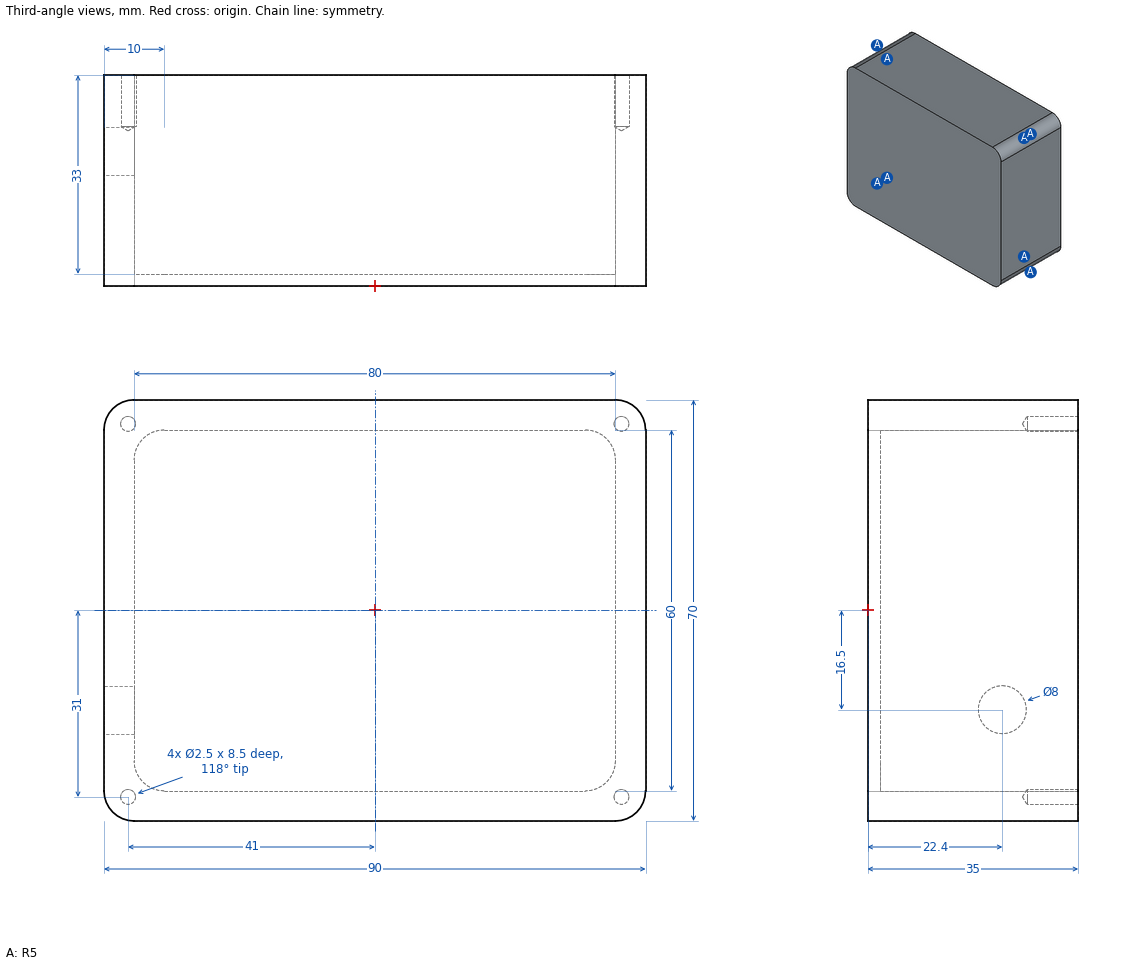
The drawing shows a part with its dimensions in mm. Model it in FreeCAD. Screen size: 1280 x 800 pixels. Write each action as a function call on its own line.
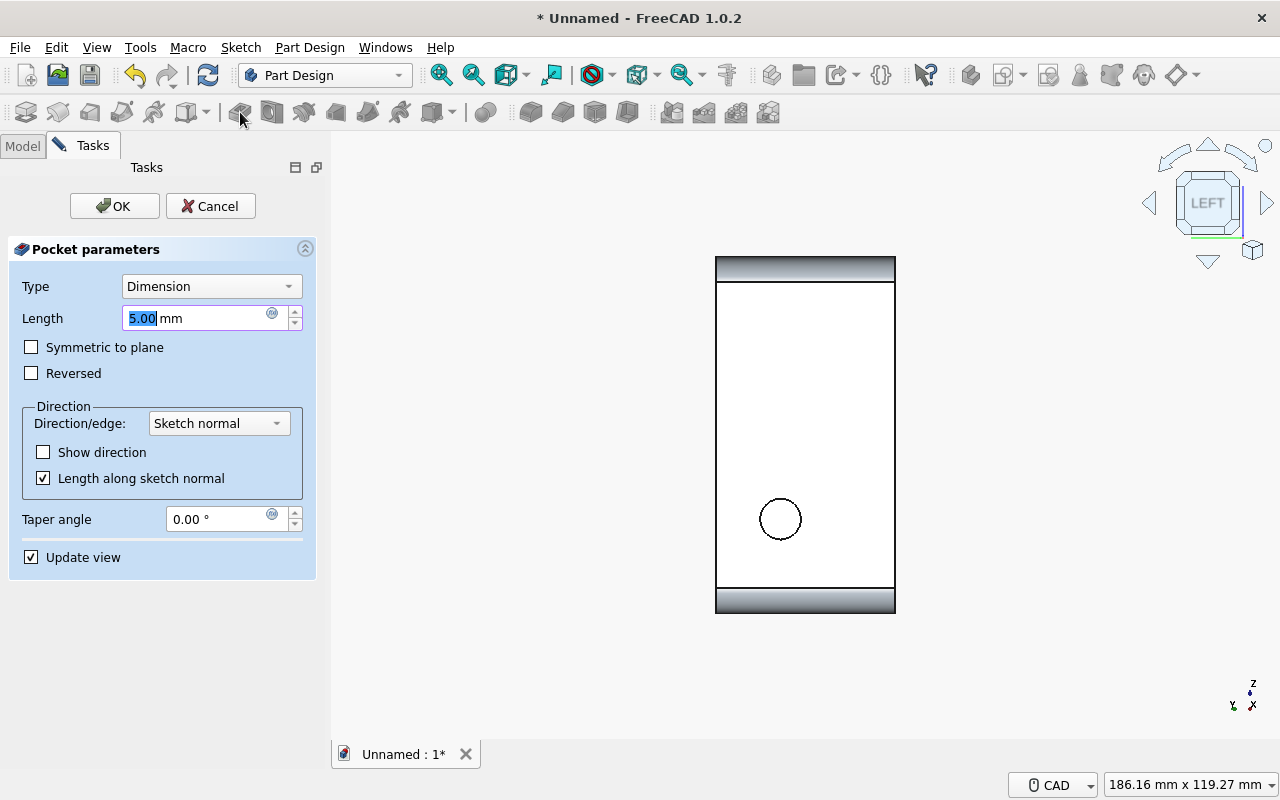
text(10)
key(Tab)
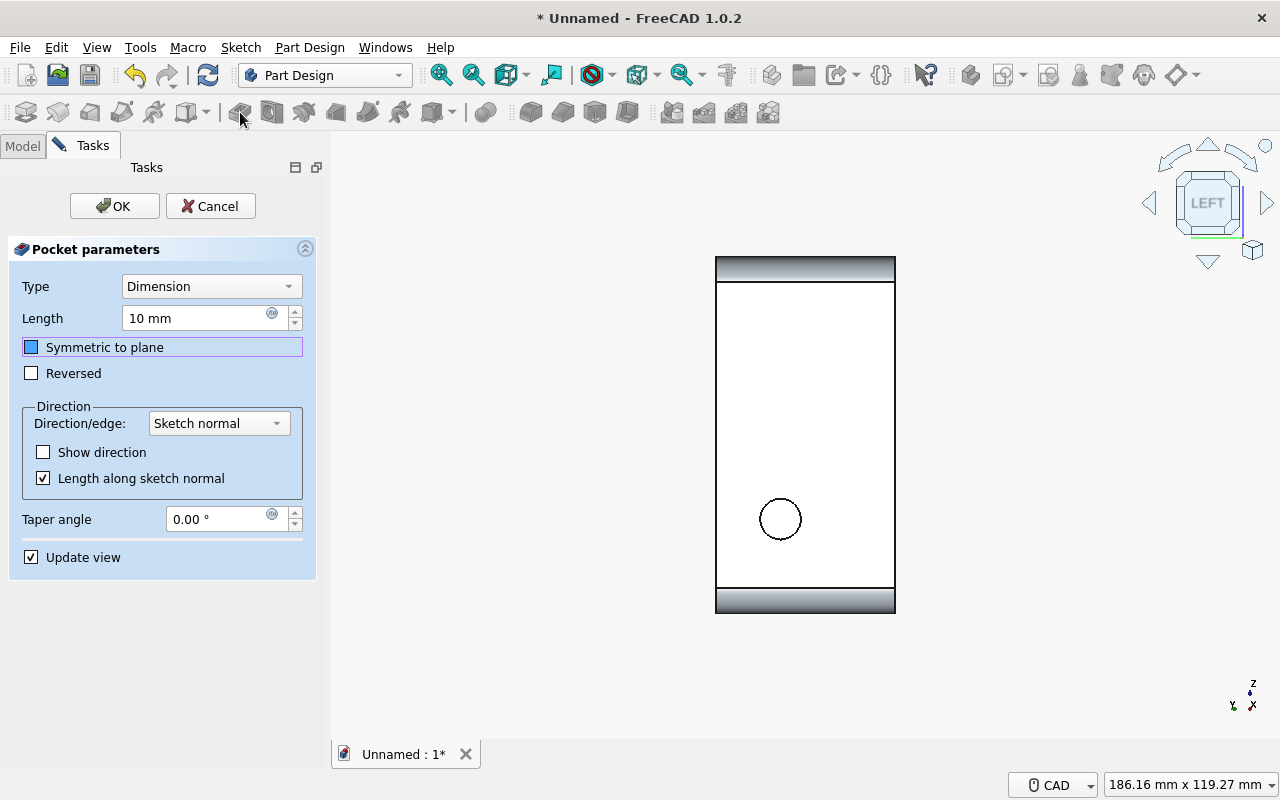
click(115, 206)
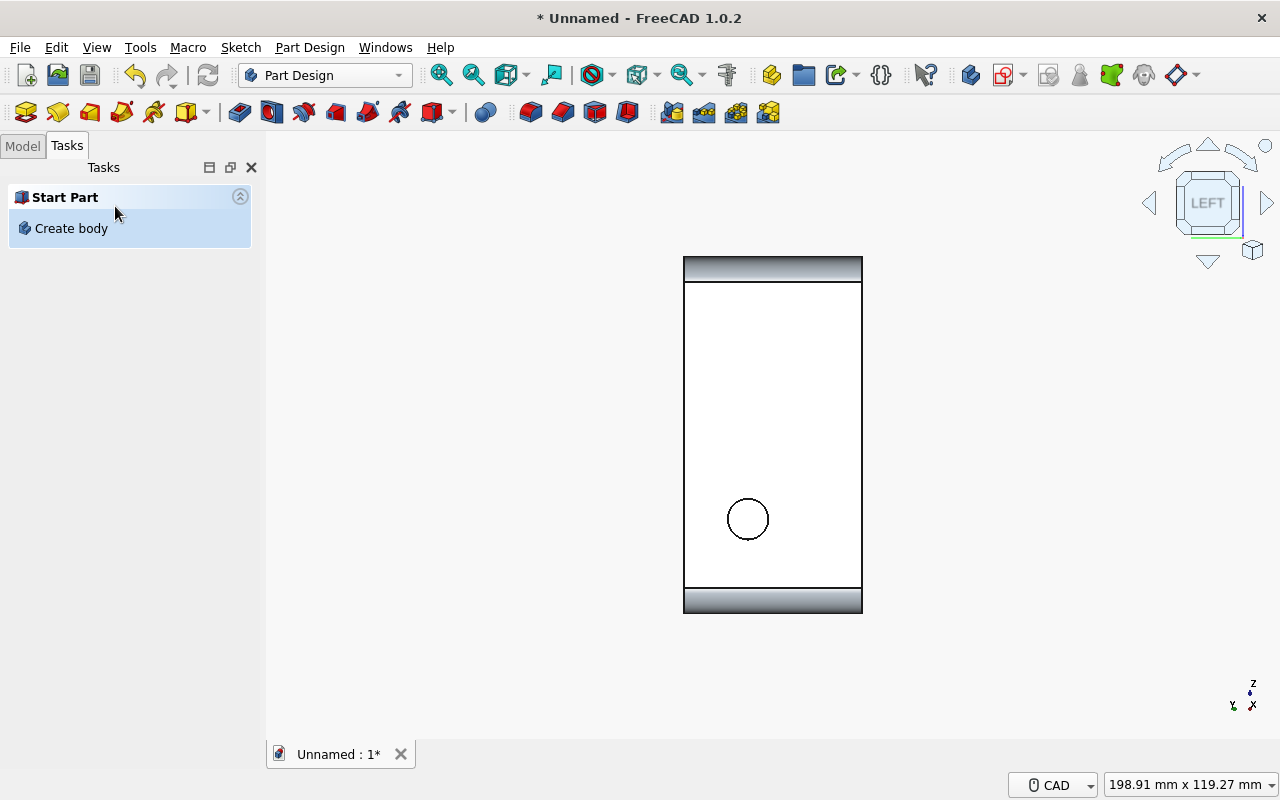
key(0)